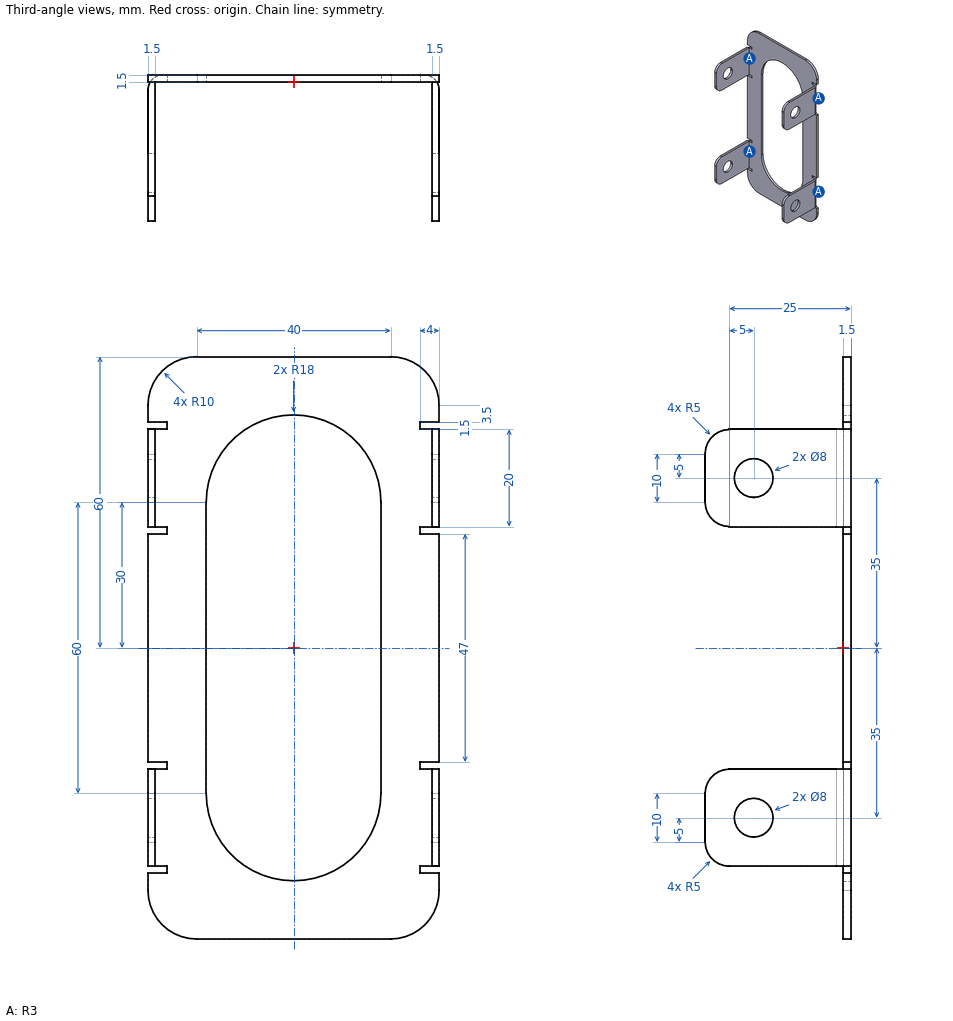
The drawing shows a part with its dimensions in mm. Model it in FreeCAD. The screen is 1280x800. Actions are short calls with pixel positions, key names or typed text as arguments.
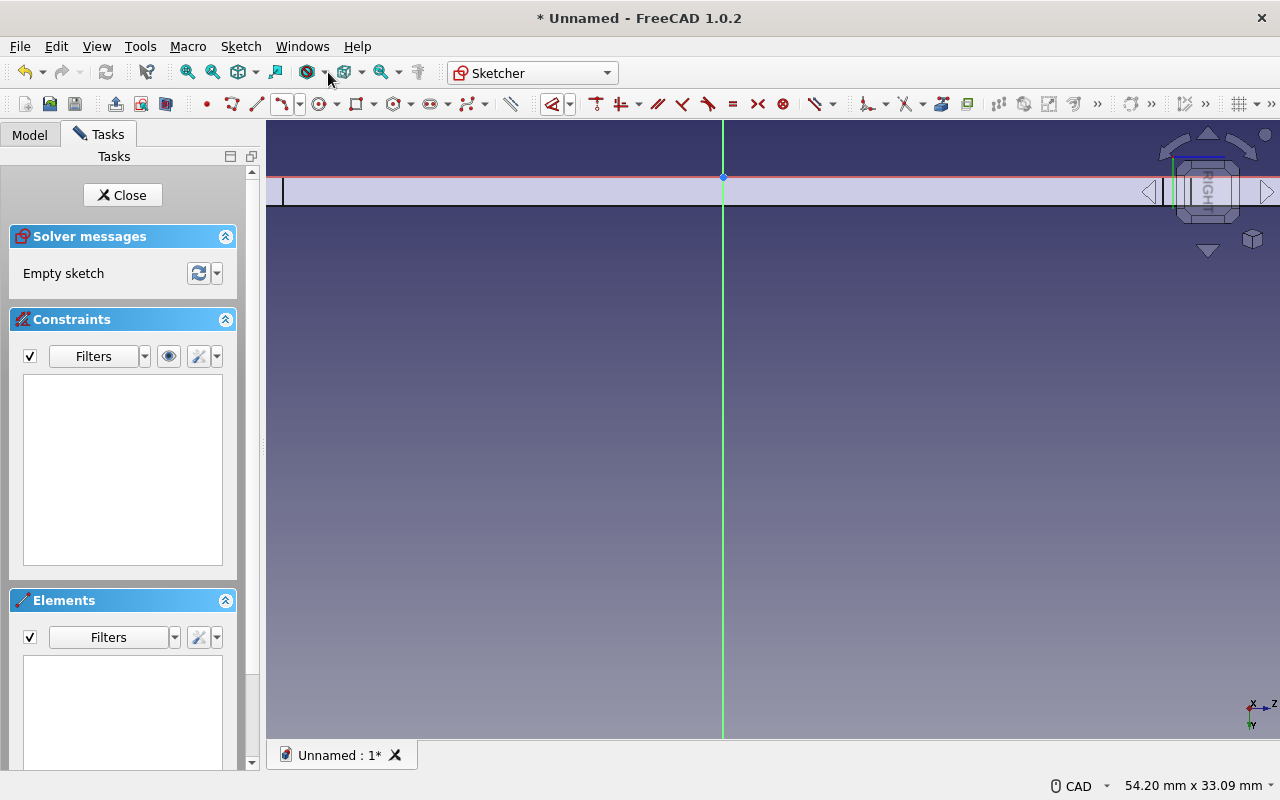
scroll(694, 711, down, 5)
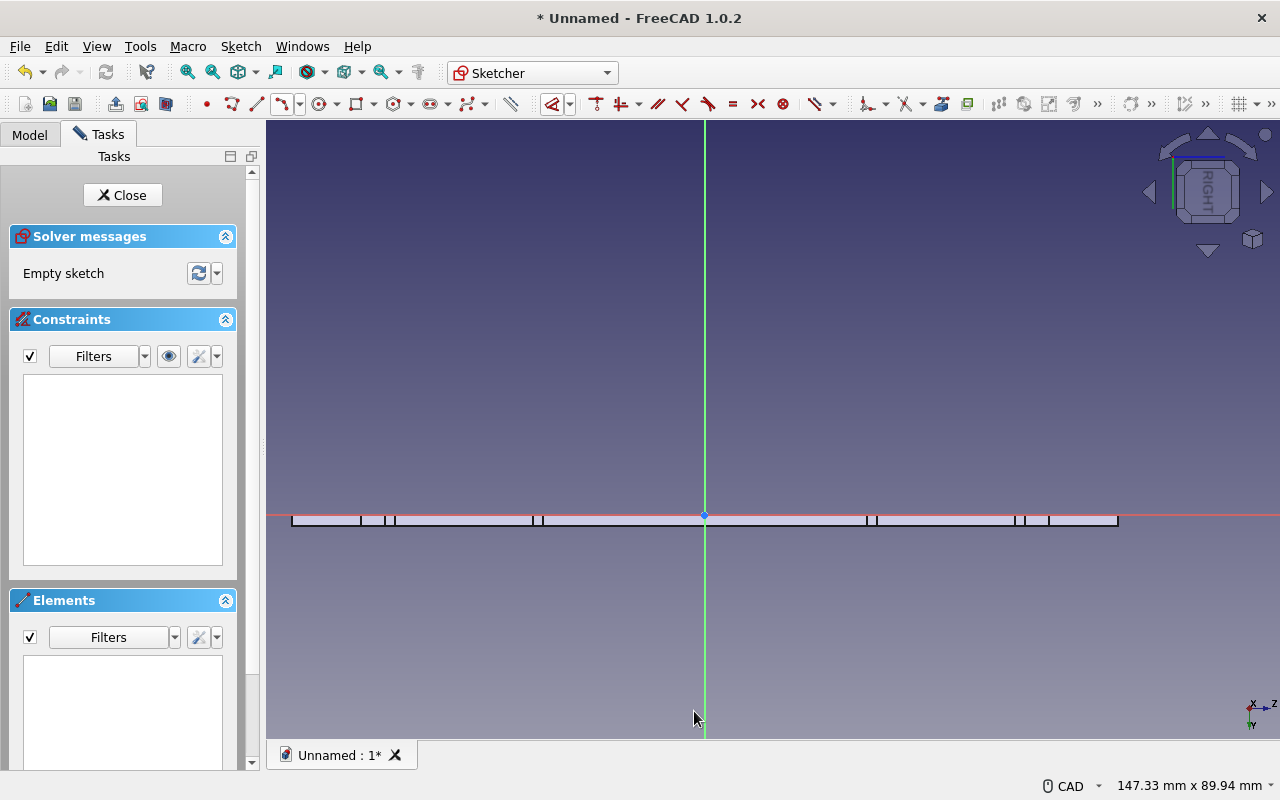
key(g)
key(l)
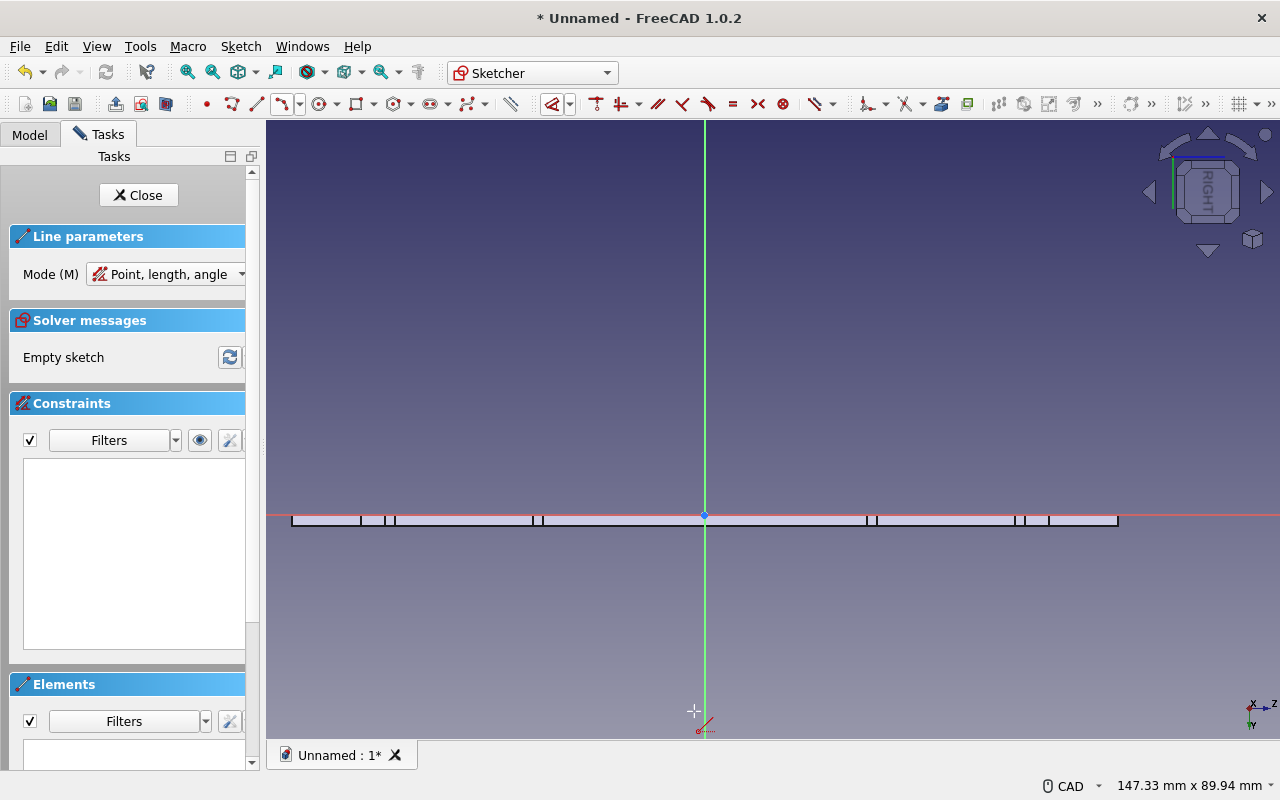
click(980, 319)
click(911, 319)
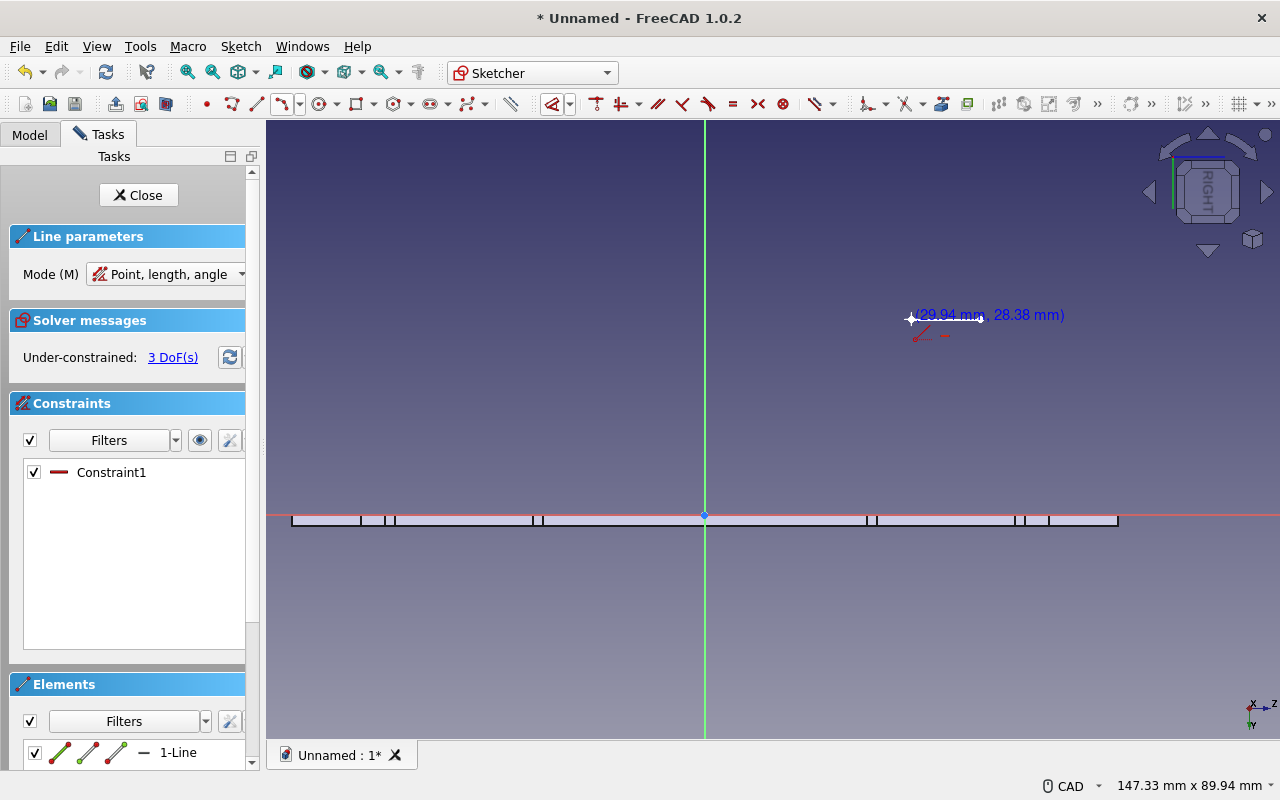
key(g)
key(m)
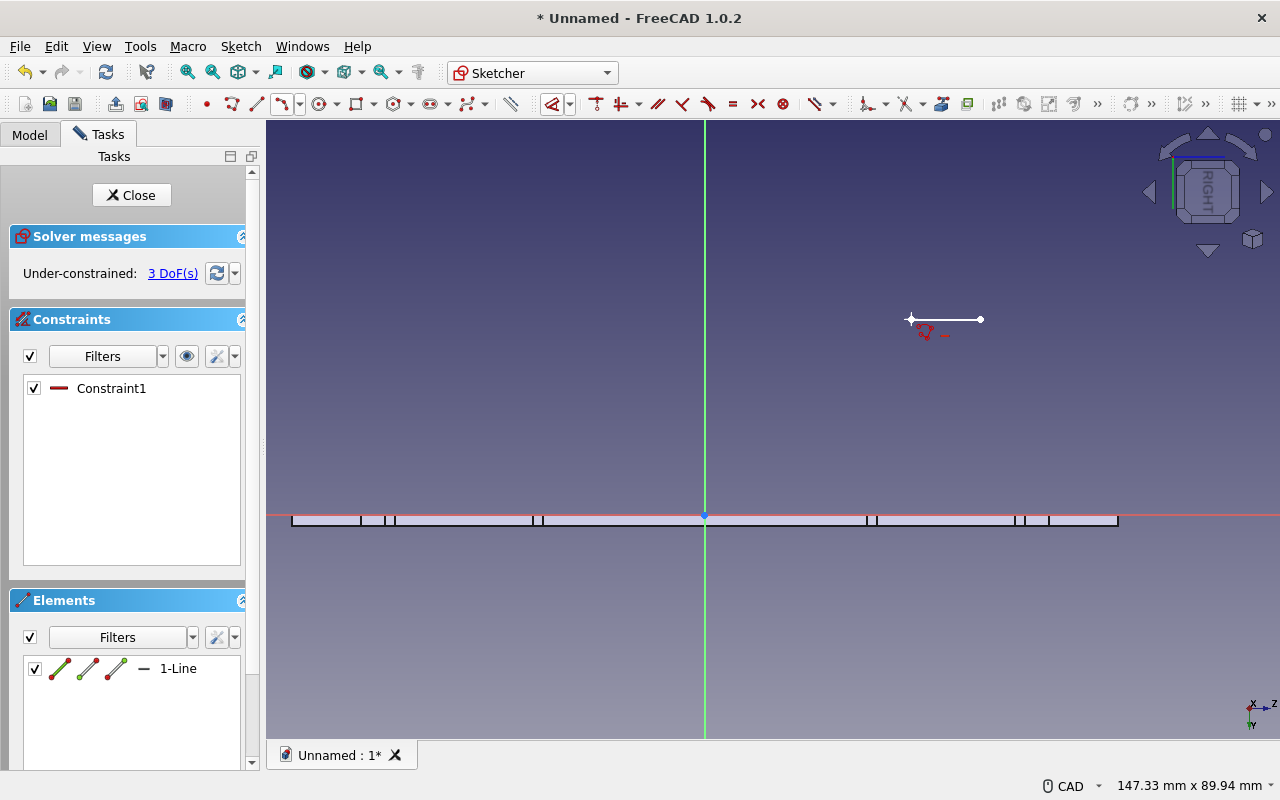
click(877, 354)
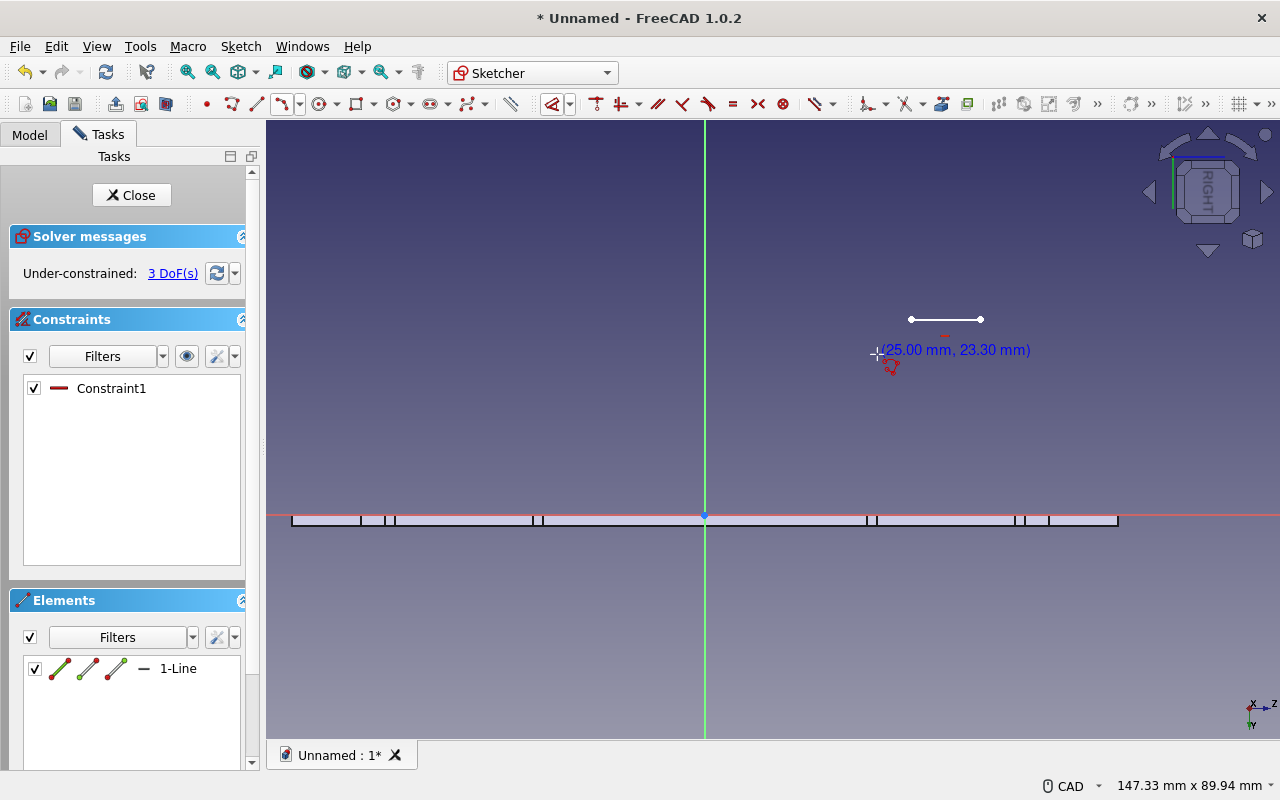
scroll(877, 526, up, 3)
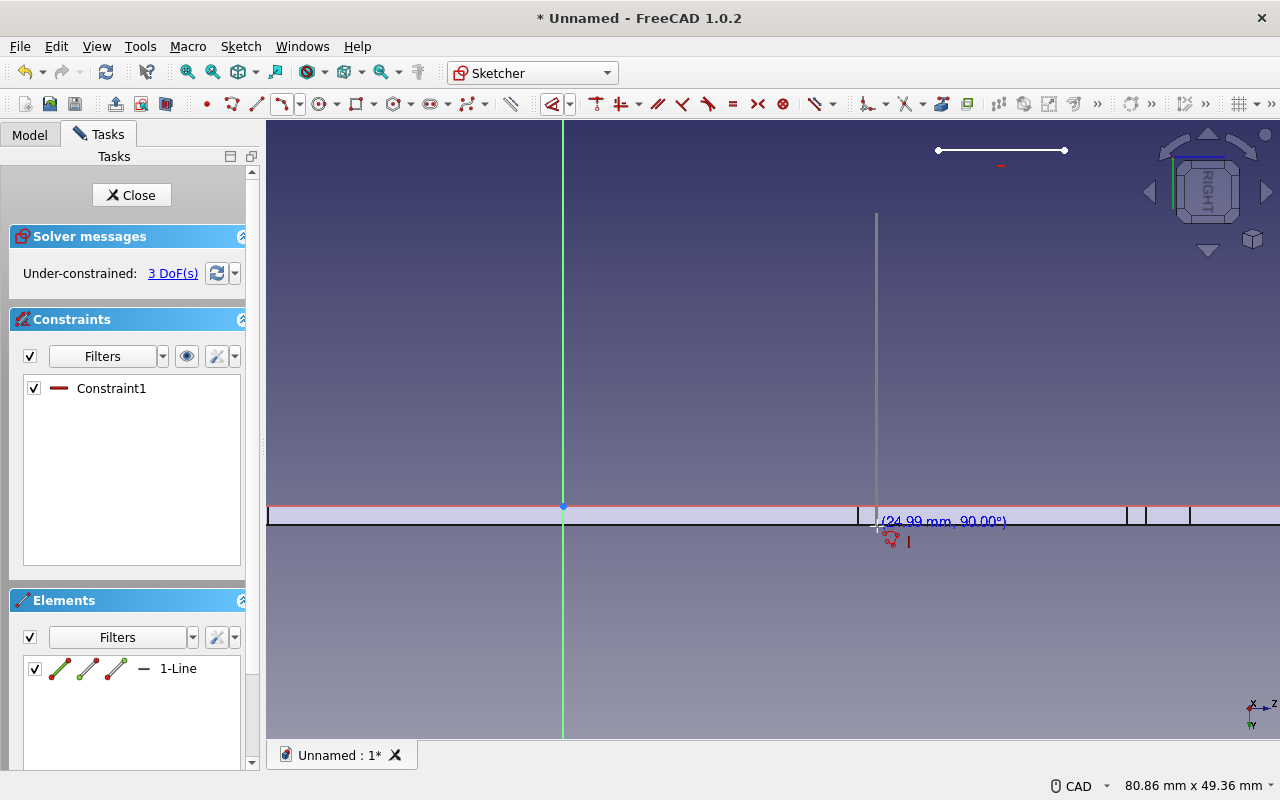
click(877, 525)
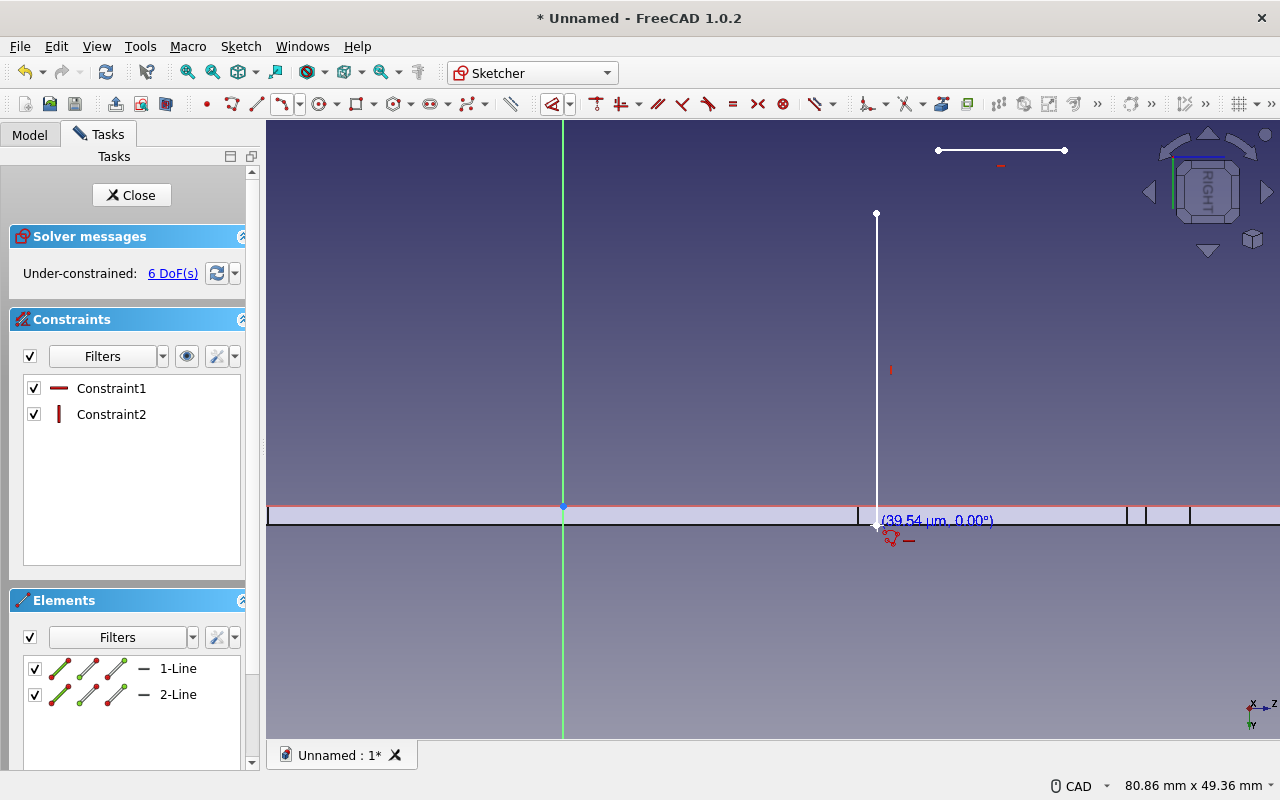
scroll(877, 542, down, 3)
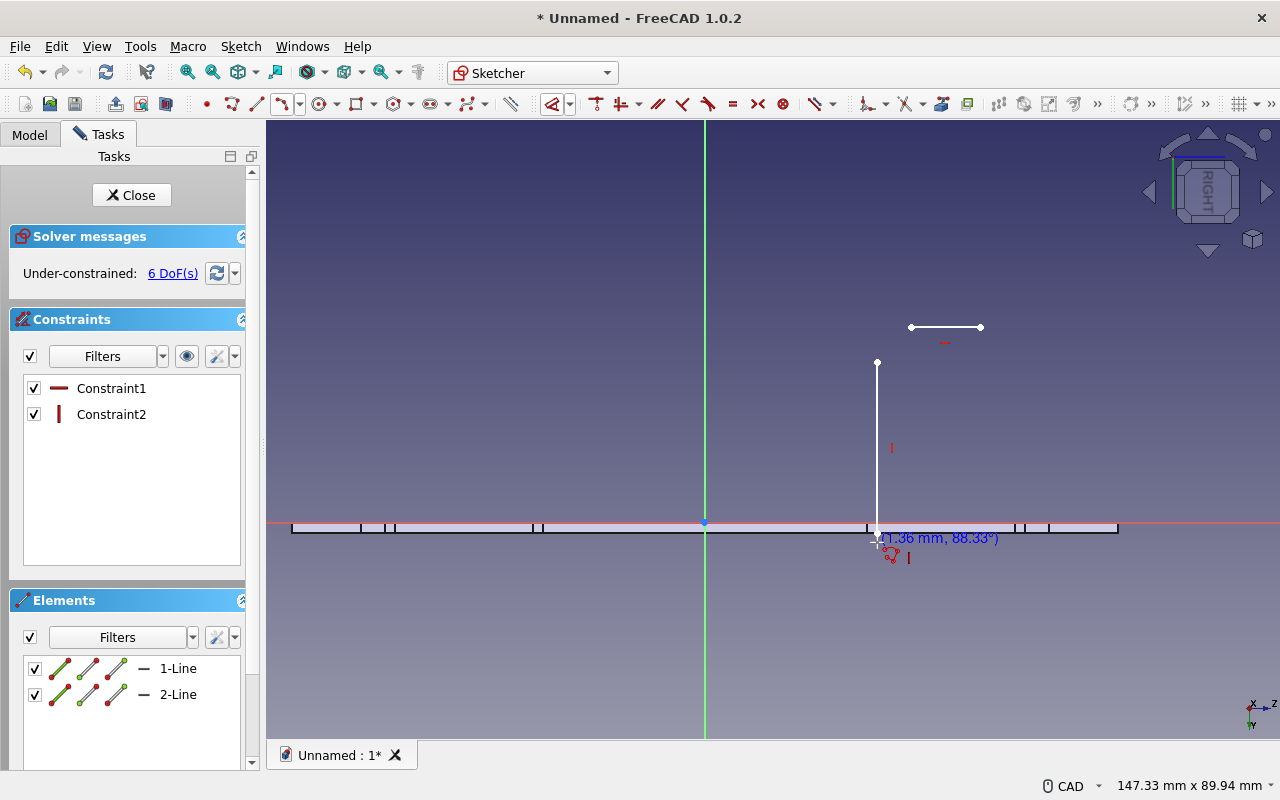
scroll(1015, 533, up, 3)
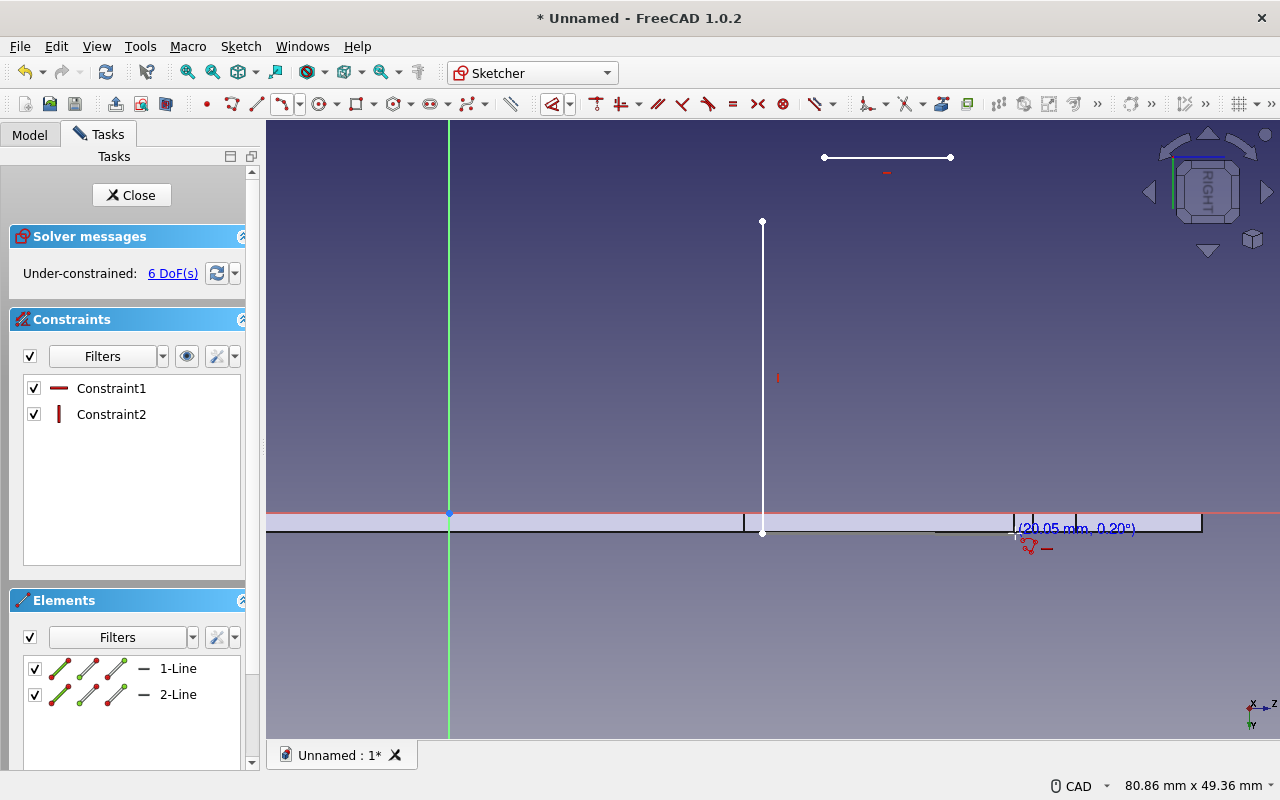
click(1014, 532)
click(1014, 219)
right_click(1014, 219)